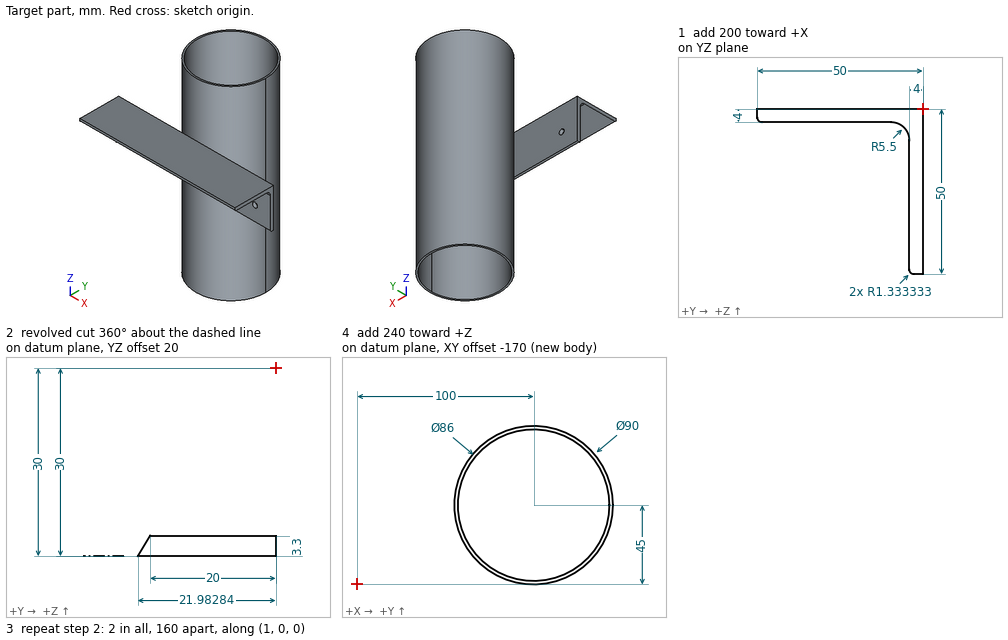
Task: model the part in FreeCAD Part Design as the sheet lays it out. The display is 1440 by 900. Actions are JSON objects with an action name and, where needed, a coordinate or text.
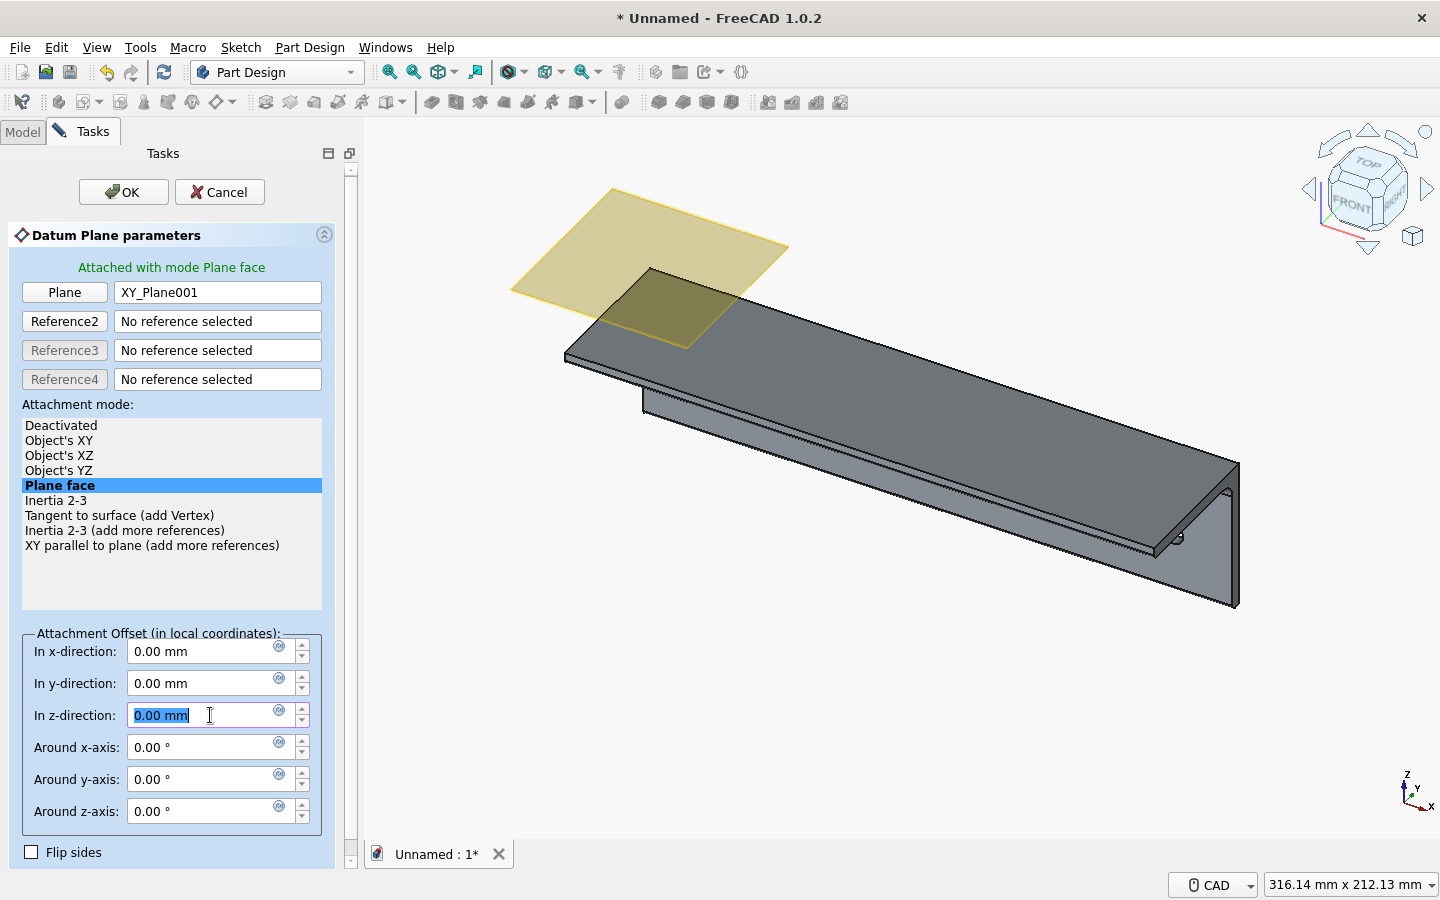
{"action": "type", "text": "-170"}
{"action": "key", "text": "Tab"}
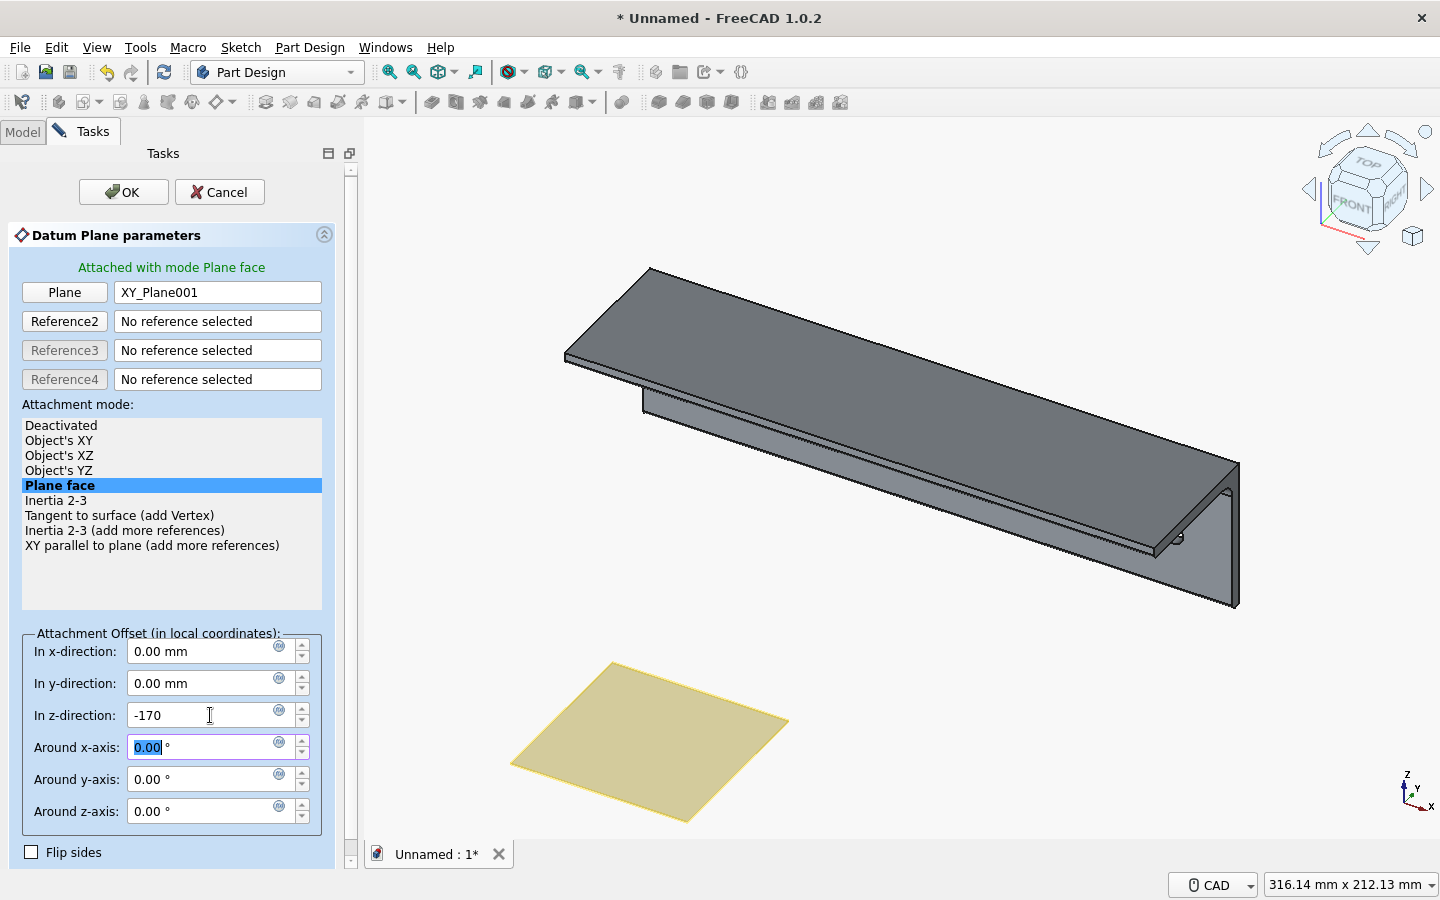
{"action": "left_click", "coordinate": [124, 192]}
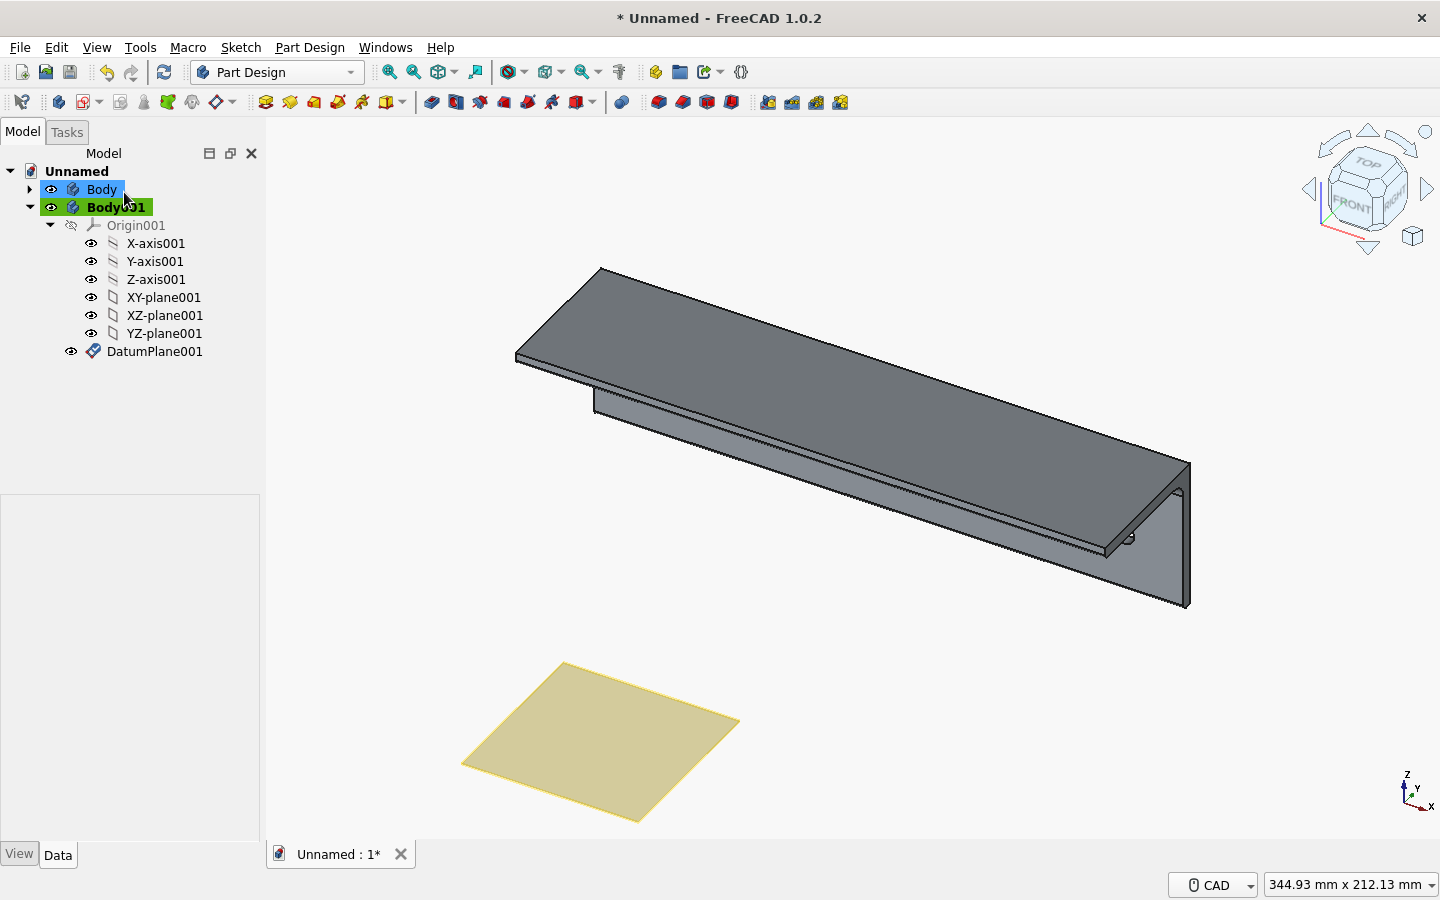
{"action": "left_click", "coordinate": [116, 351]}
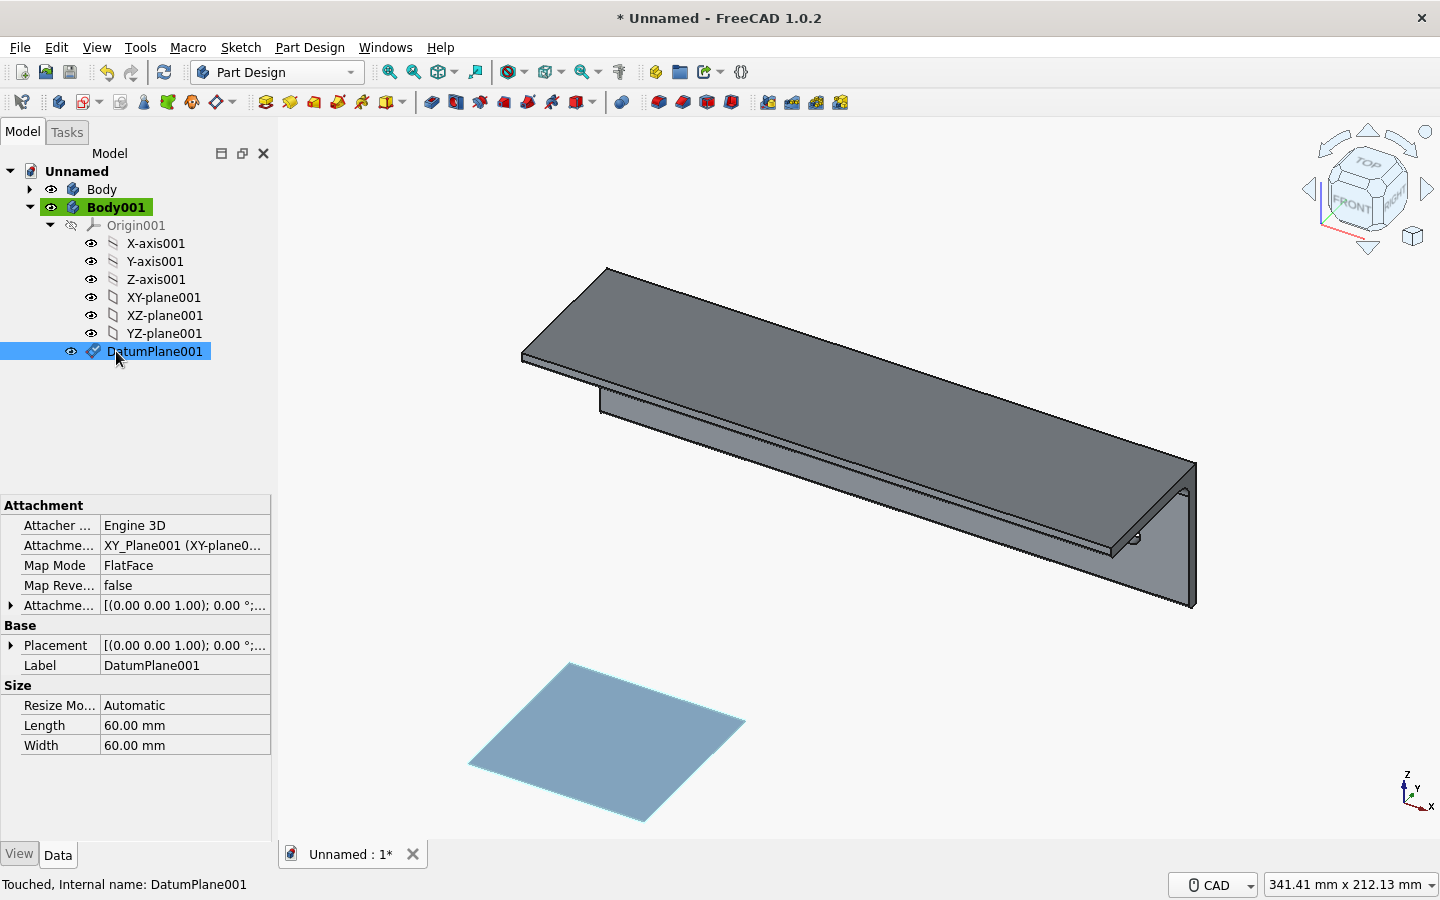
{"action": "left_click", "coordinate": [84, 102]}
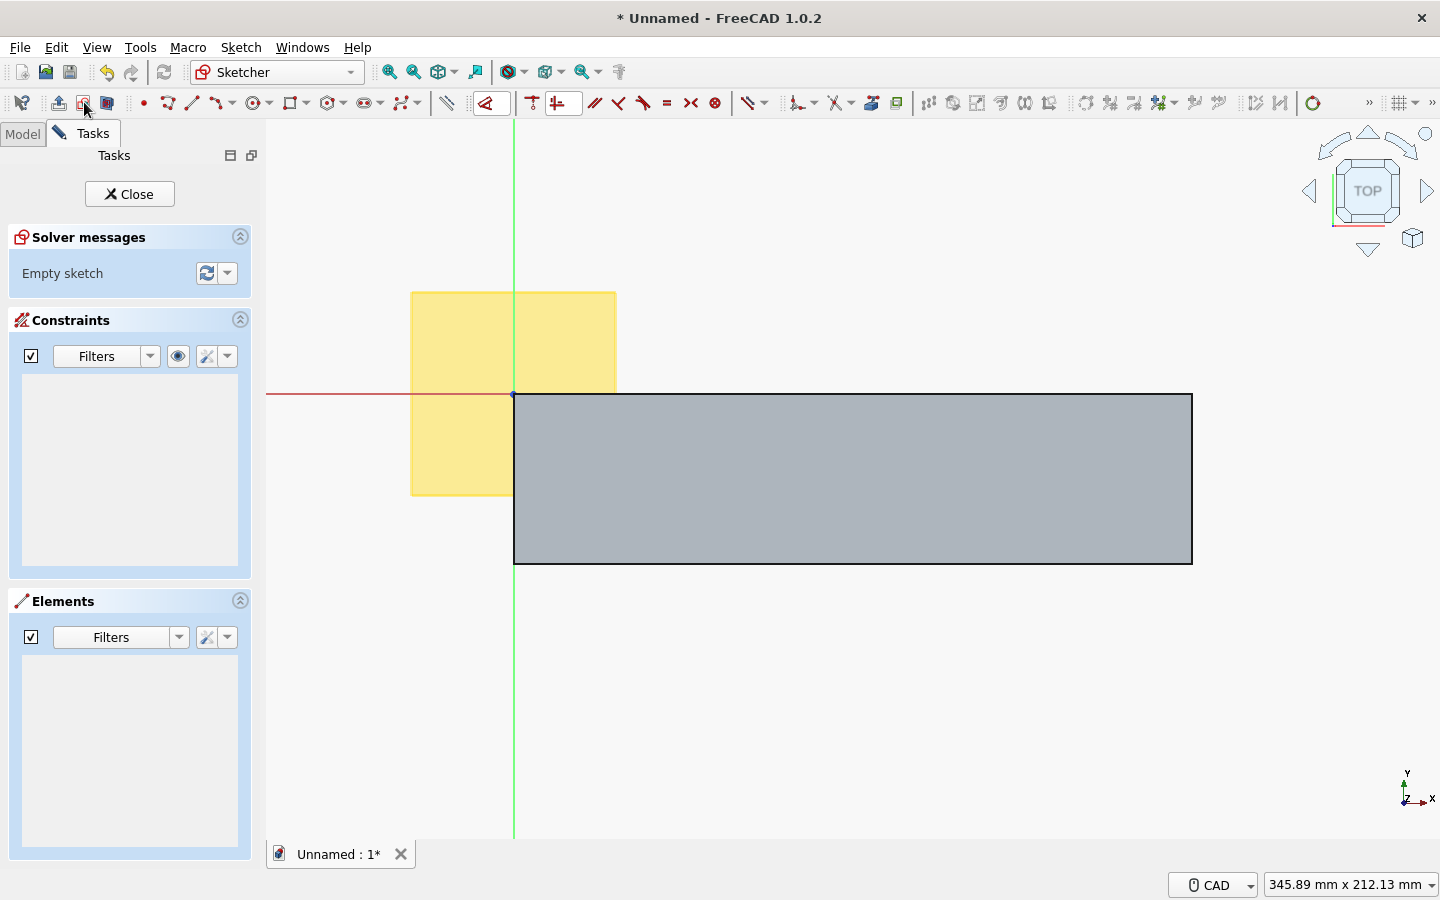
{"action": "scroll", "coordinate": [897, 811], "scroll_direction": "down", "scroll_amount": 1}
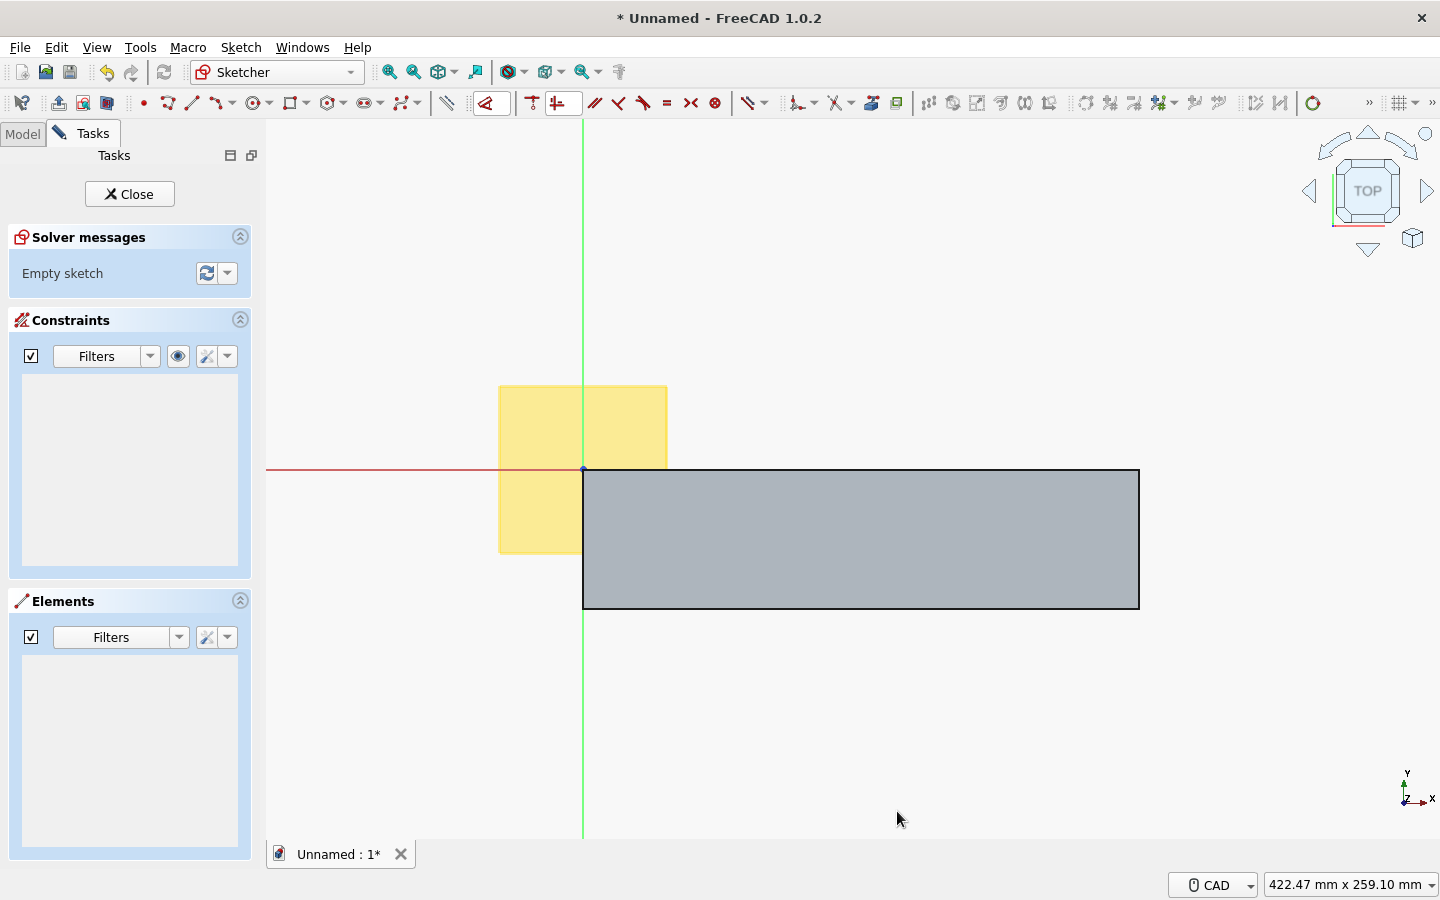
{"action": "scroll", "coordinate": [785, 182], "scroll_direction": "up", "scroll_amount": 3}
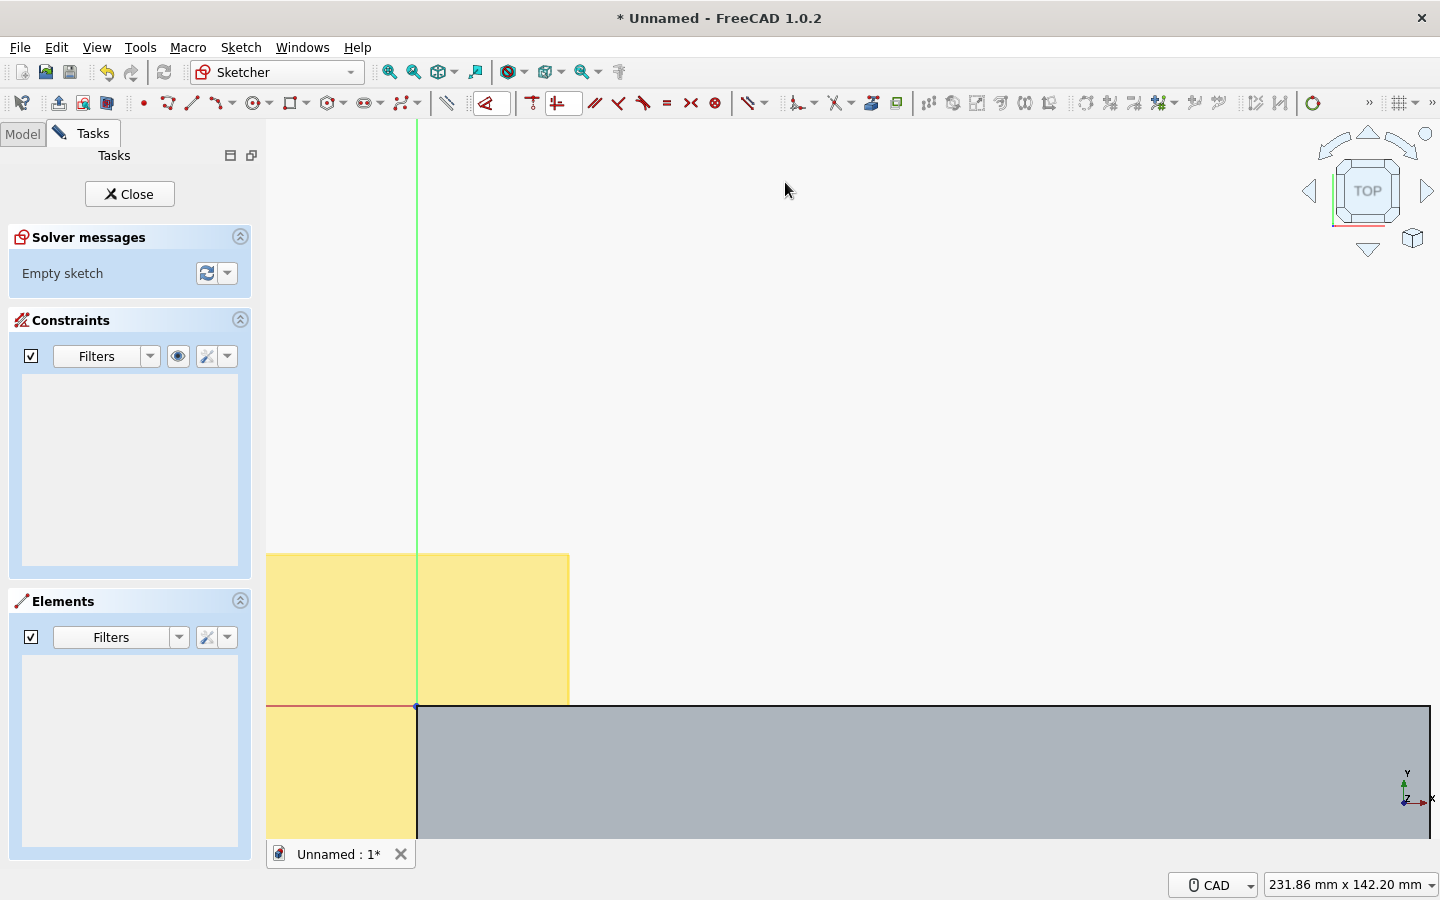
{"action": "left_click", "coordinate": [254, 104]}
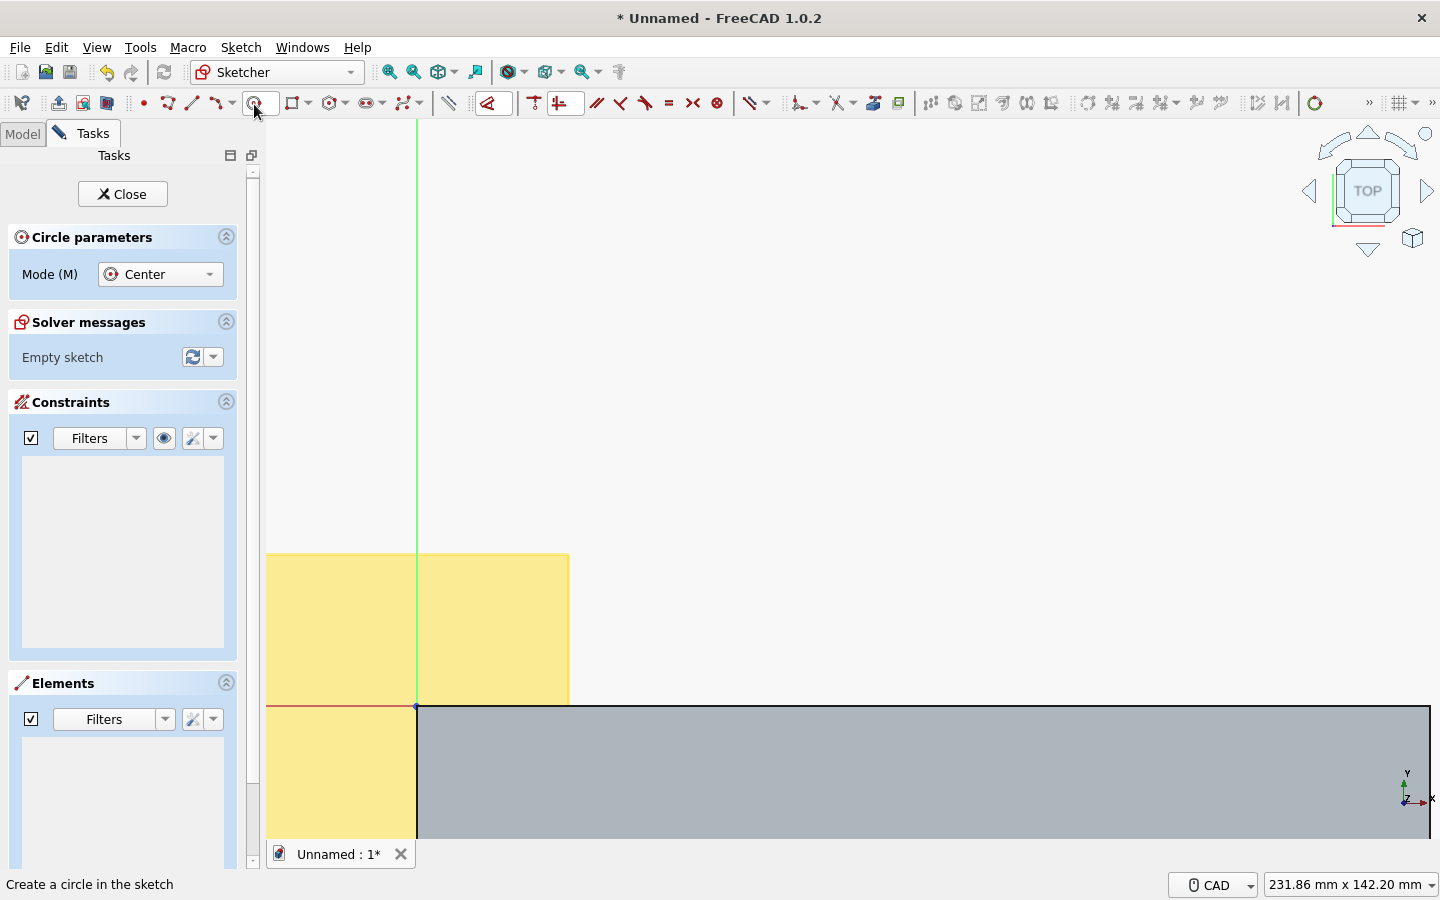
{"action": "left_click", "coordinate": [923, 479]}
{"action": "mouse_move", "coordinate": [1084, 318]}